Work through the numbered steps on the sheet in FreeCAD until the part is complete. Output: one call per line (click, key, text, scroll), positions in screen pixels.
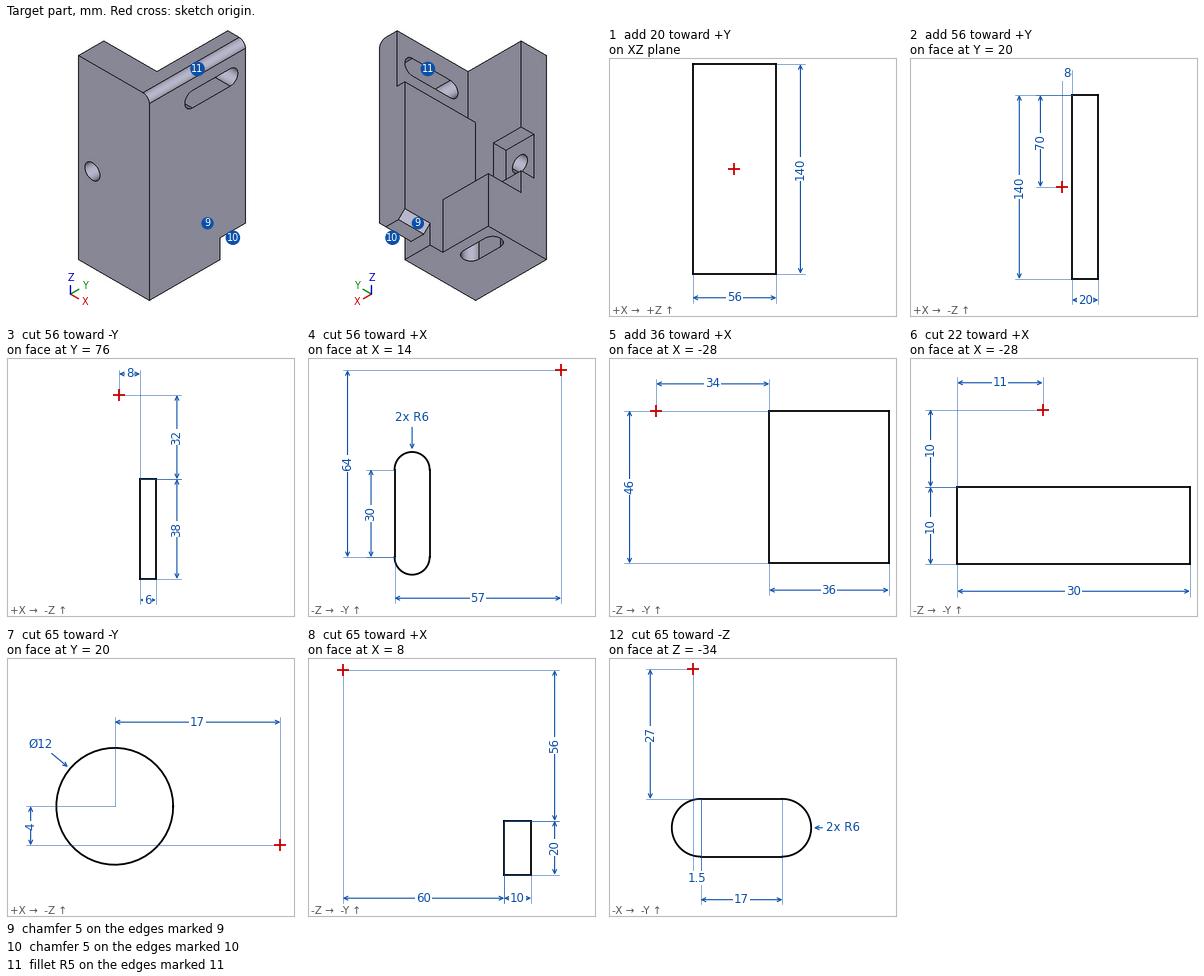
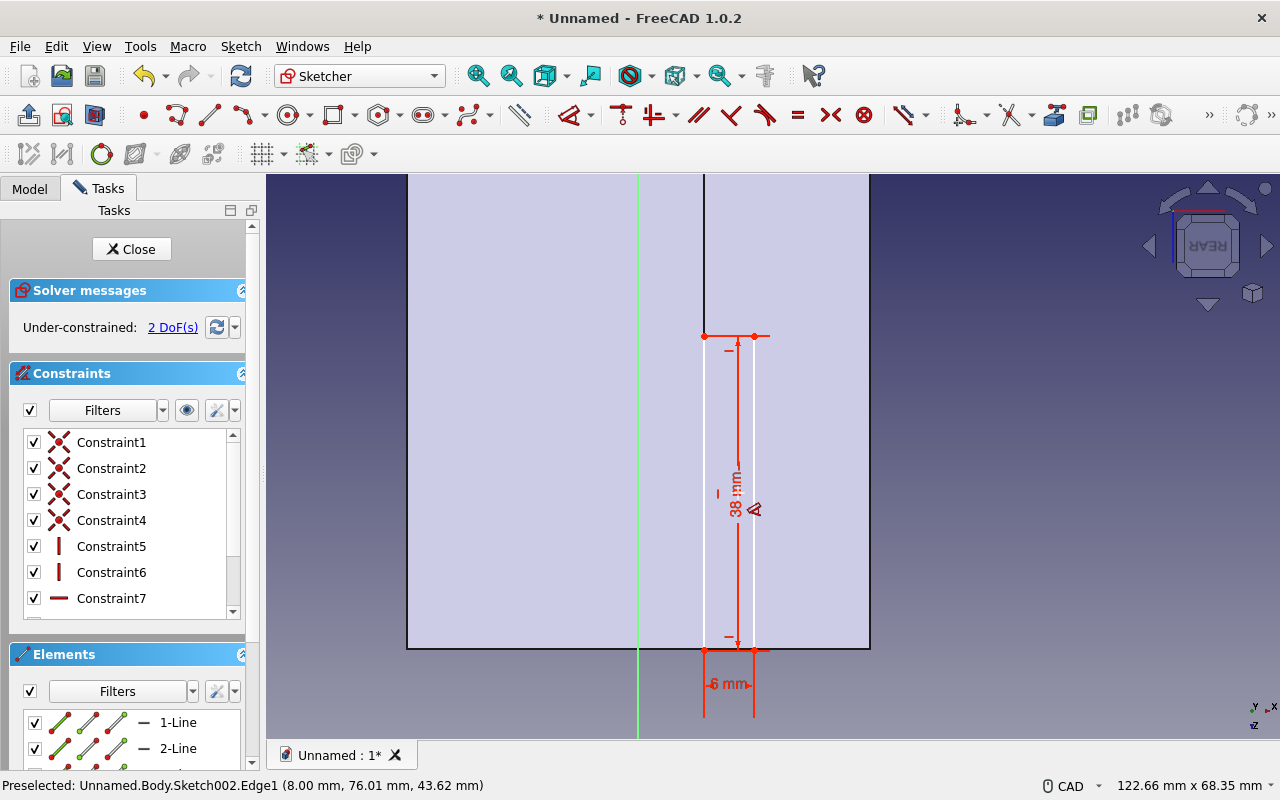
click(704, 336)
click(671, 370)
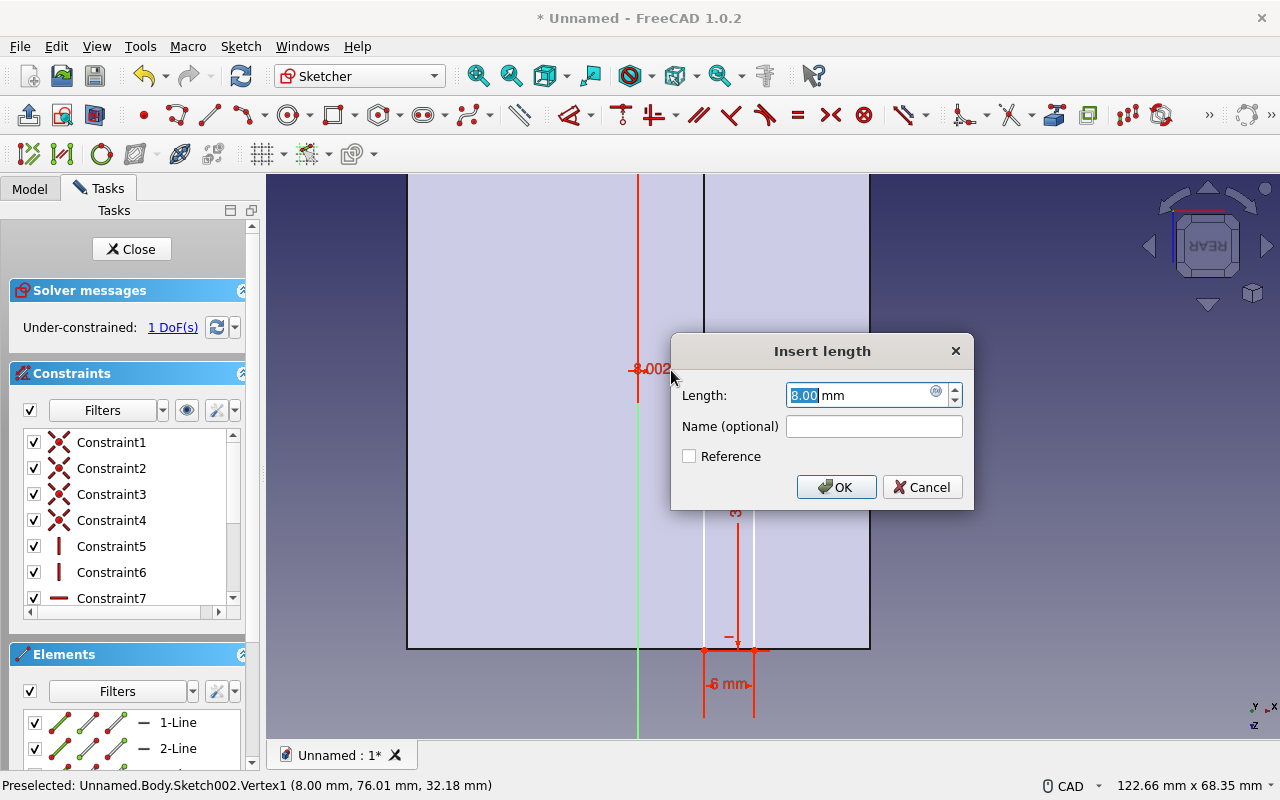
text(8)
key(Return)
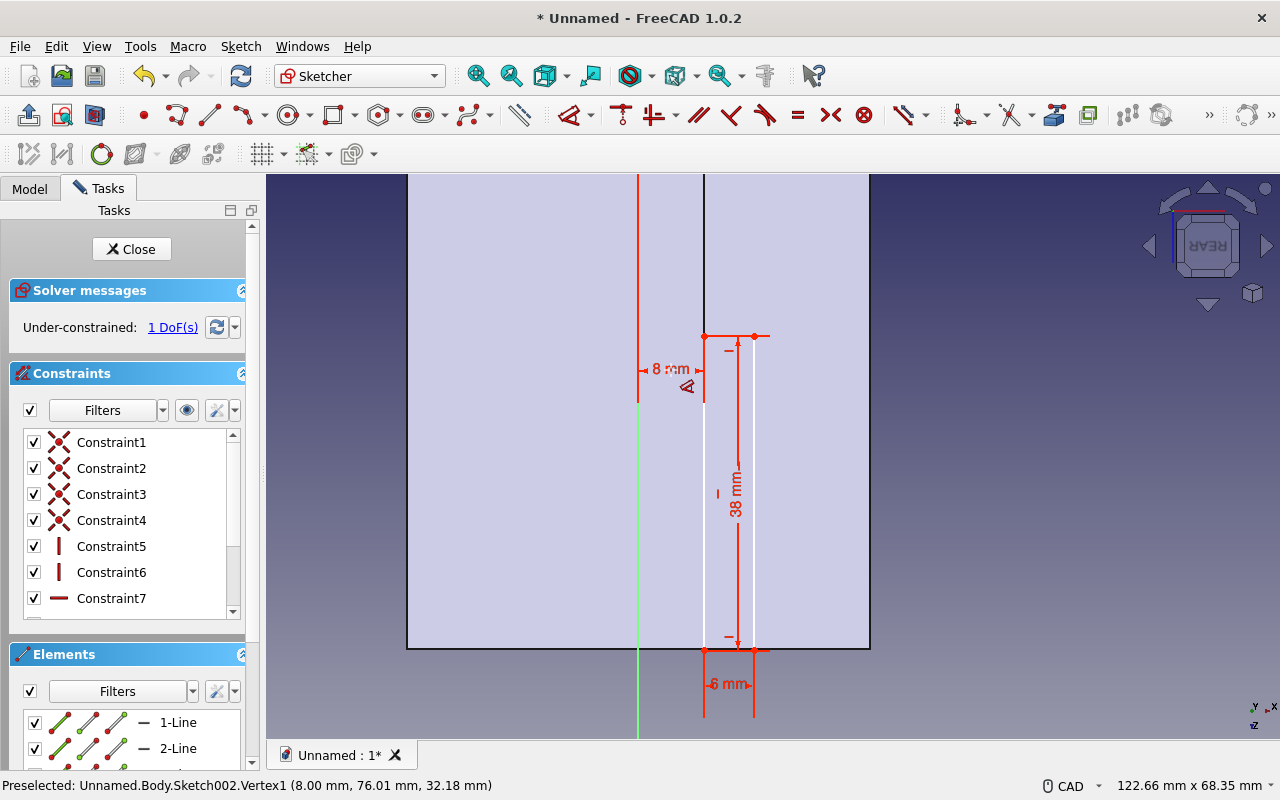
click(704, 336)
click(604, 269)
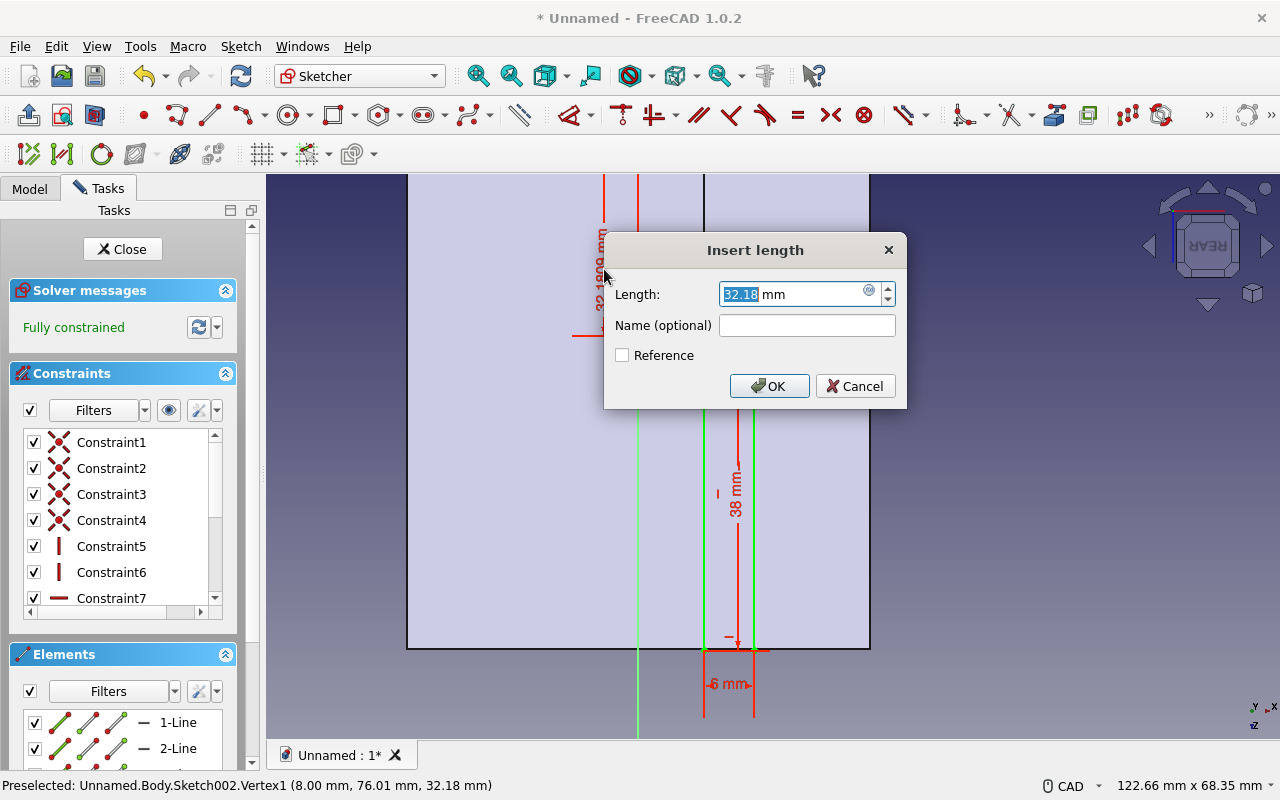
text(32)
key(Return)
key(Escape)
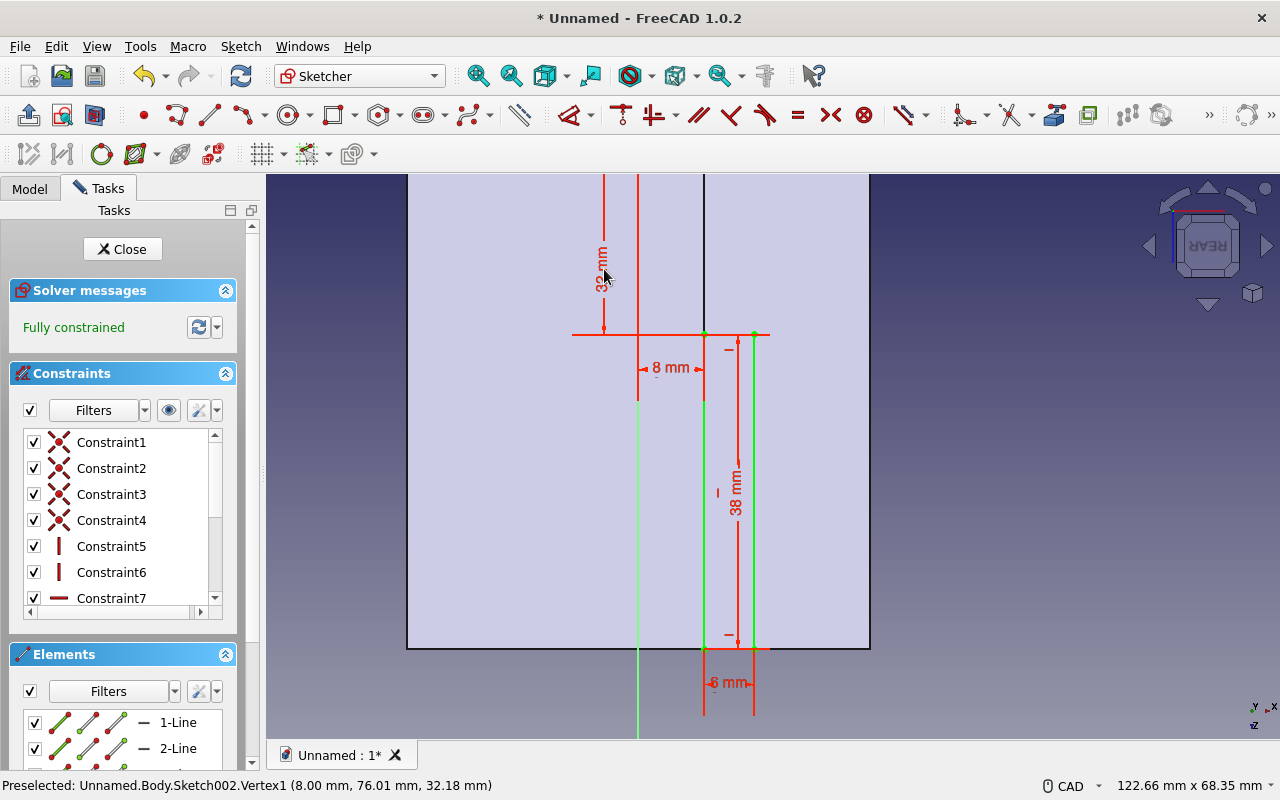
click(123, 249)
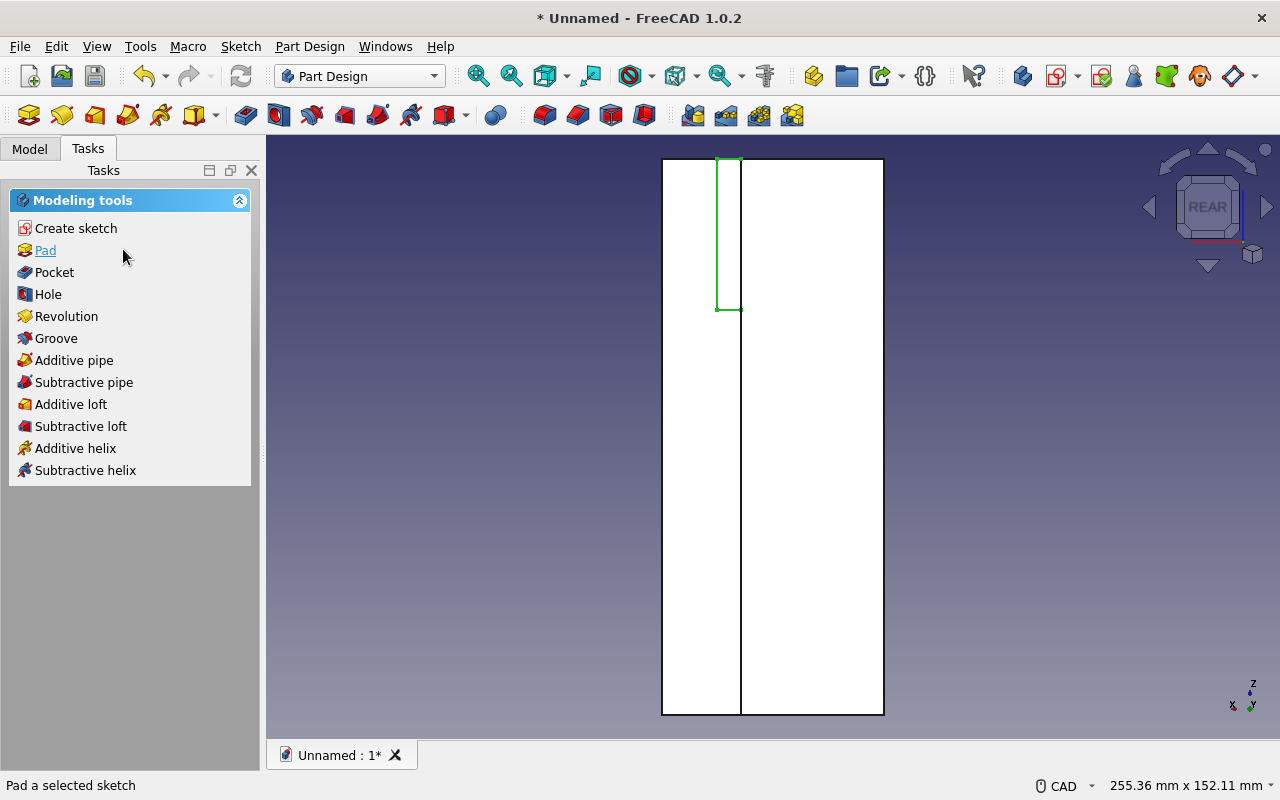
click(246, 116)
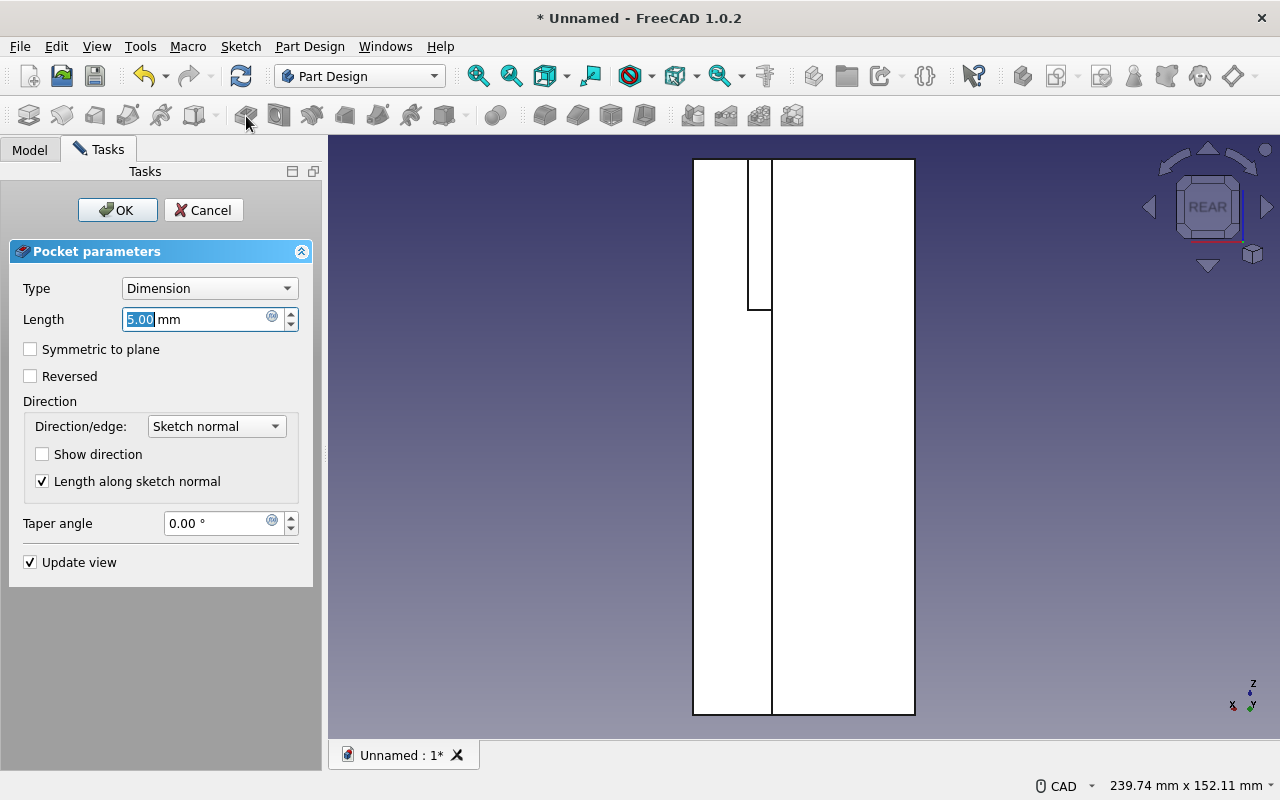
text(56)
key(Tab)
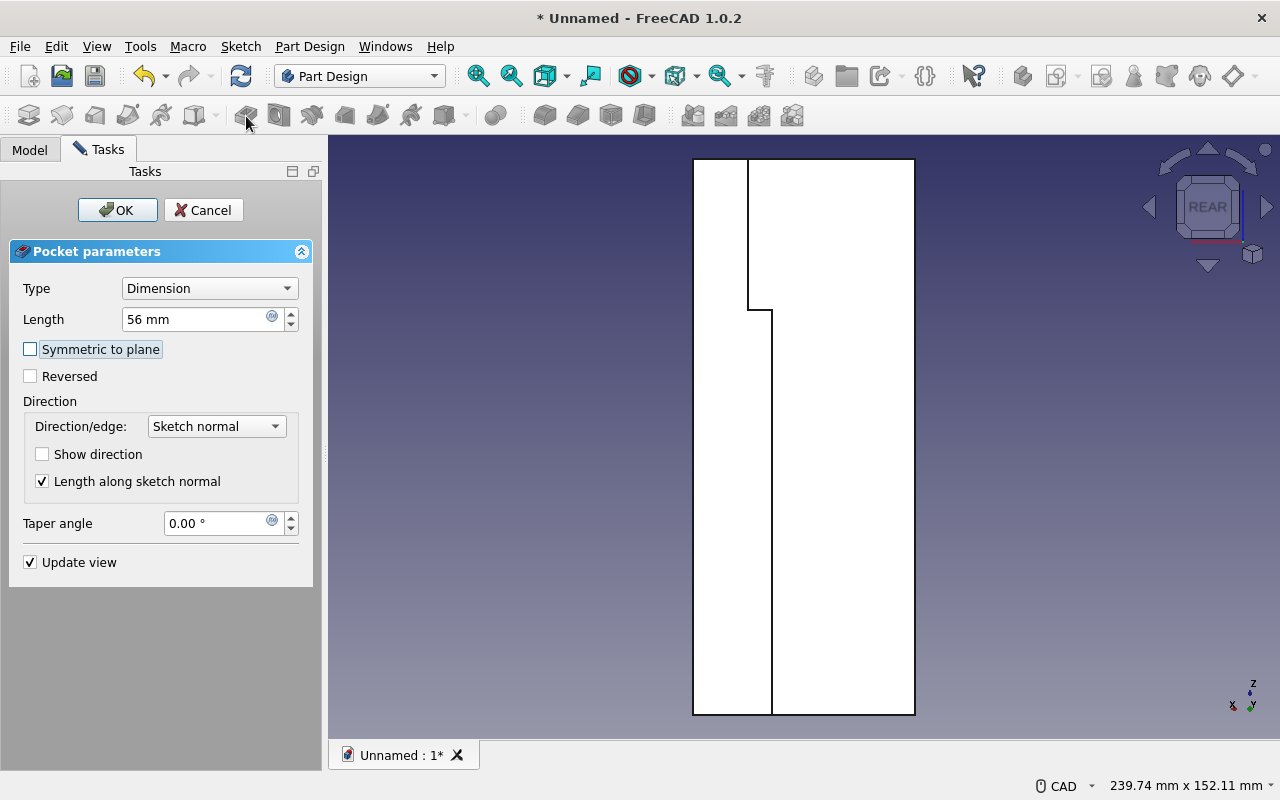
click(118, 210)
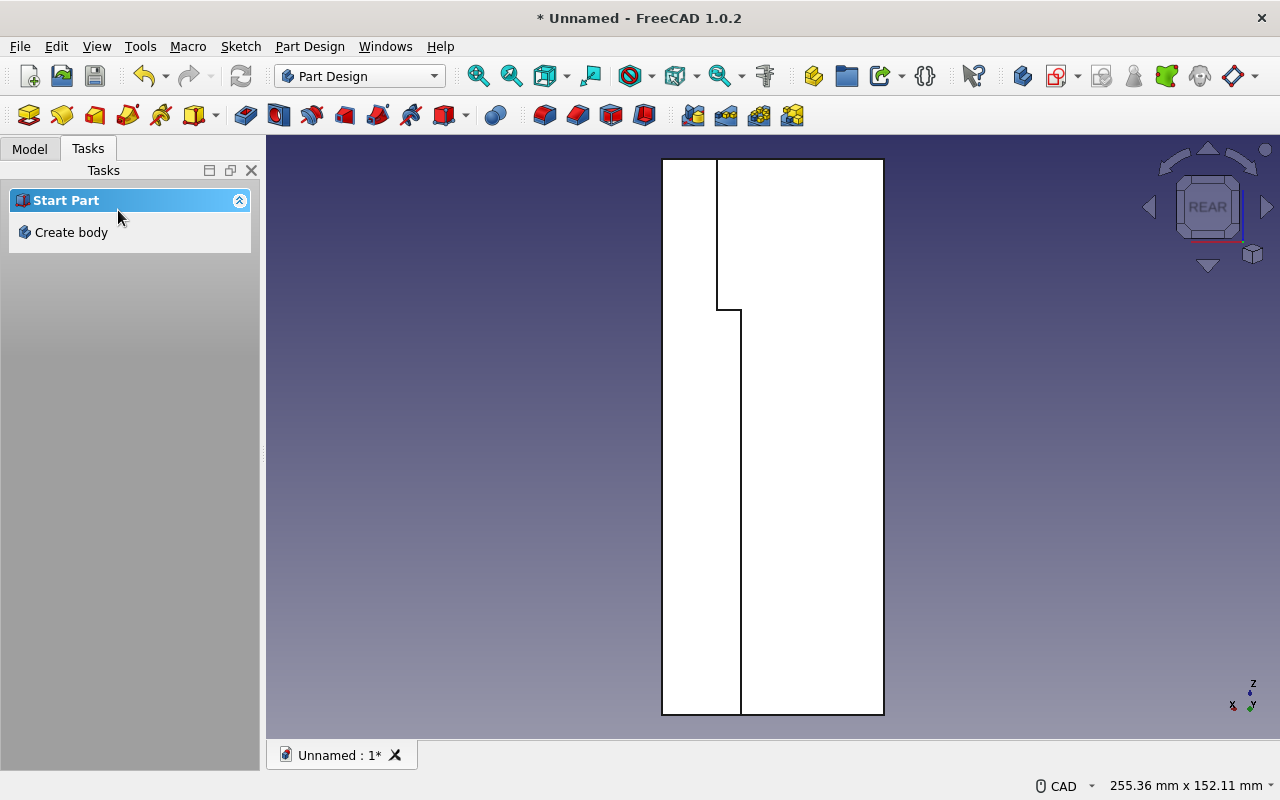
key(6)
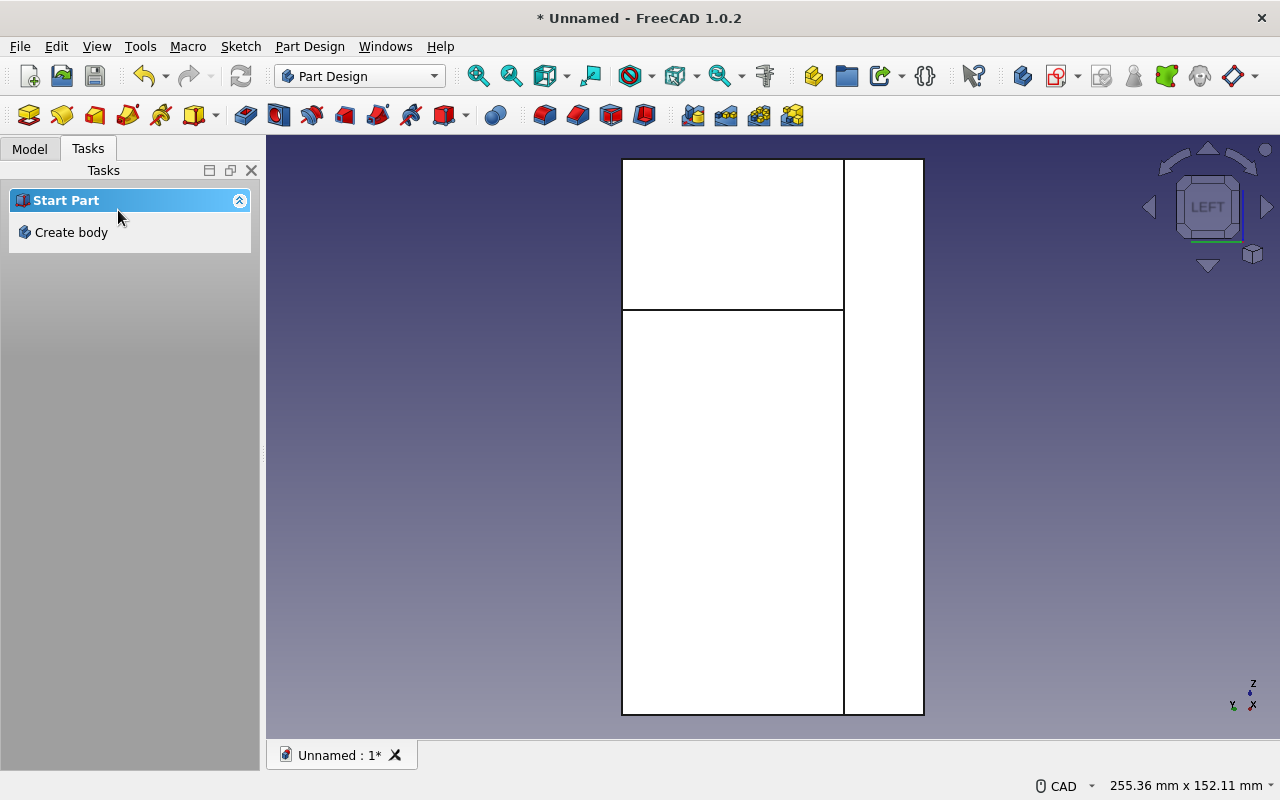
click(702, 233)